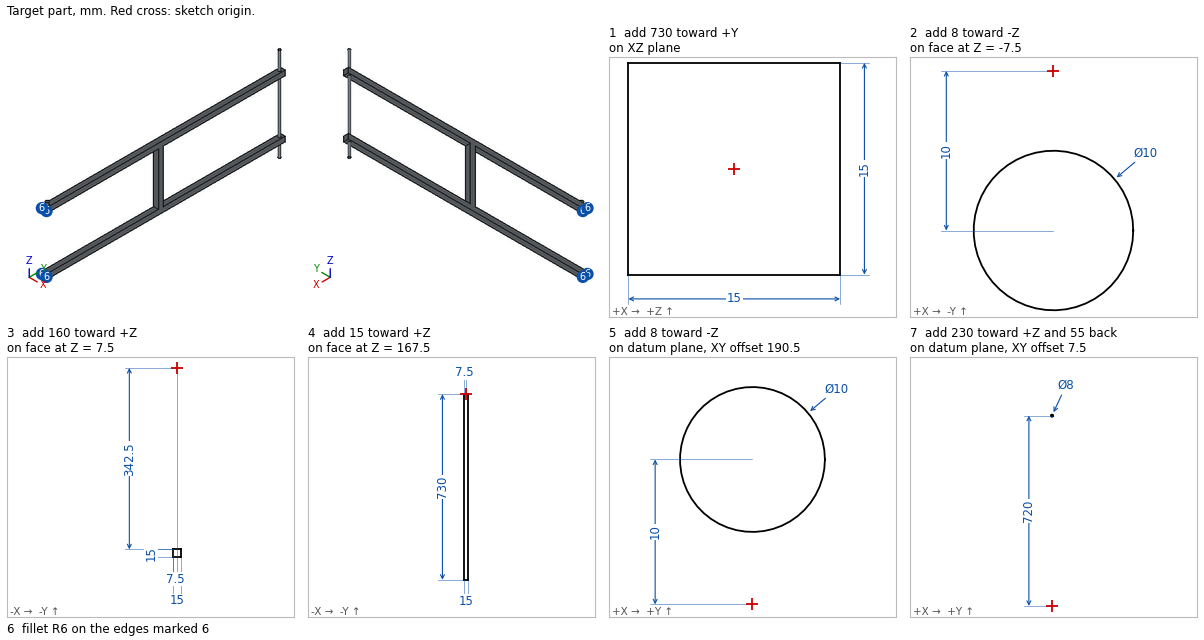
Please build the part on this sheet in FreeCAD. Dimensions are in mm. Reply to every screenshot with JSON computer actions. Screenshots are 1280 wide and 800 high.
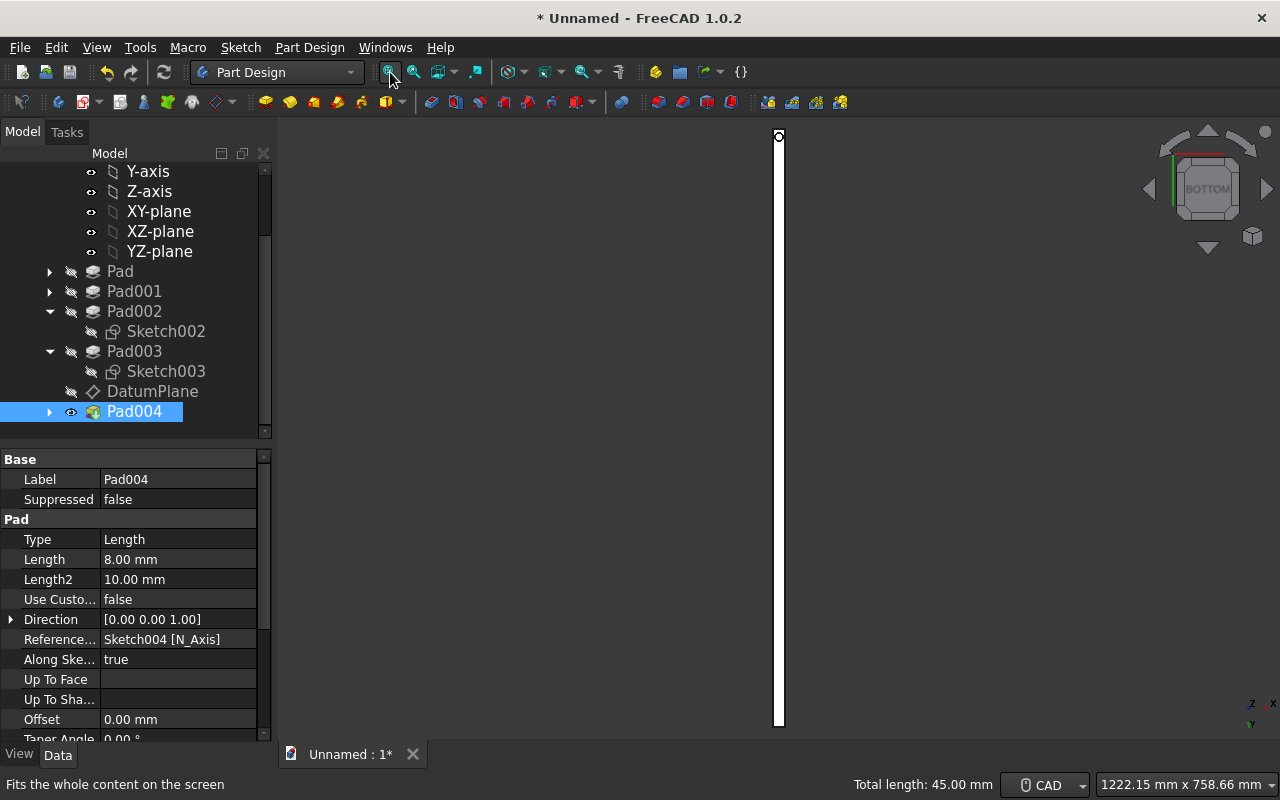
{"action": "key", "text": "4"}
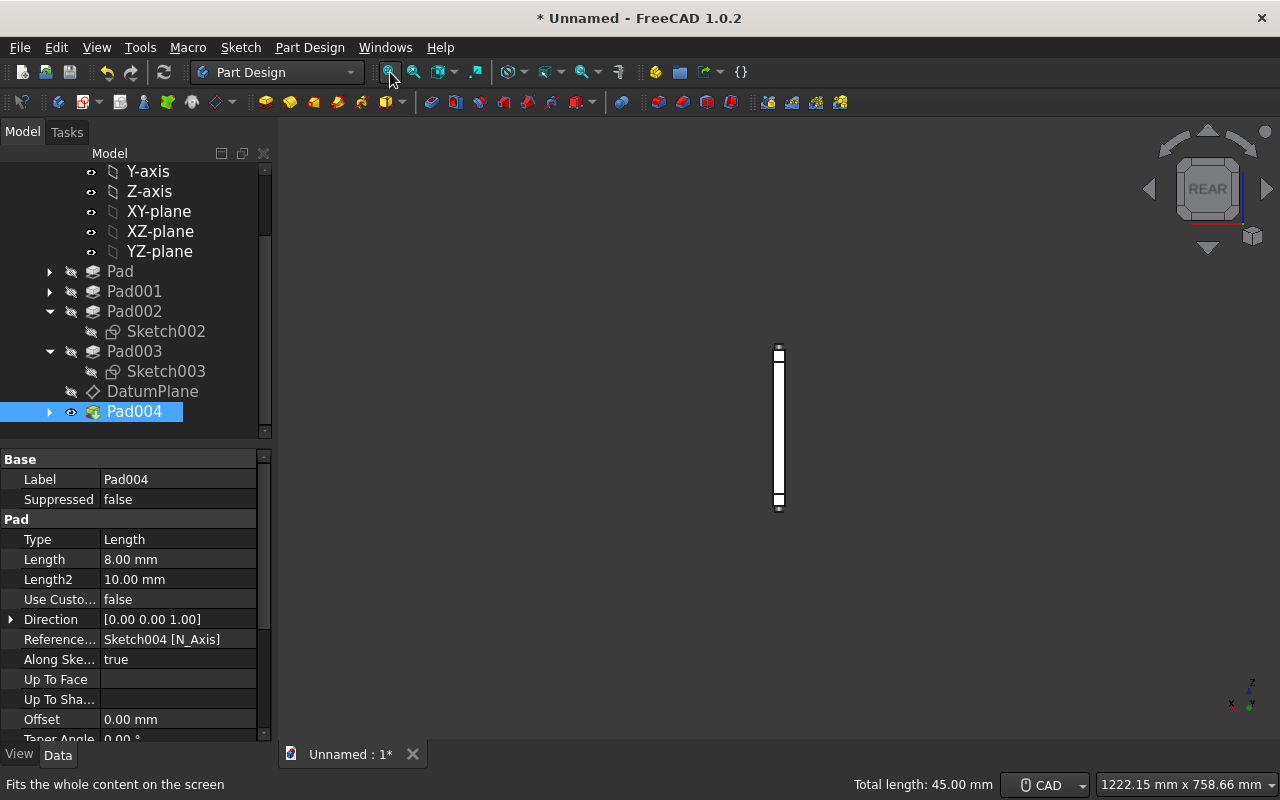
{"action": "left_click", "coordinate": [390, 72]}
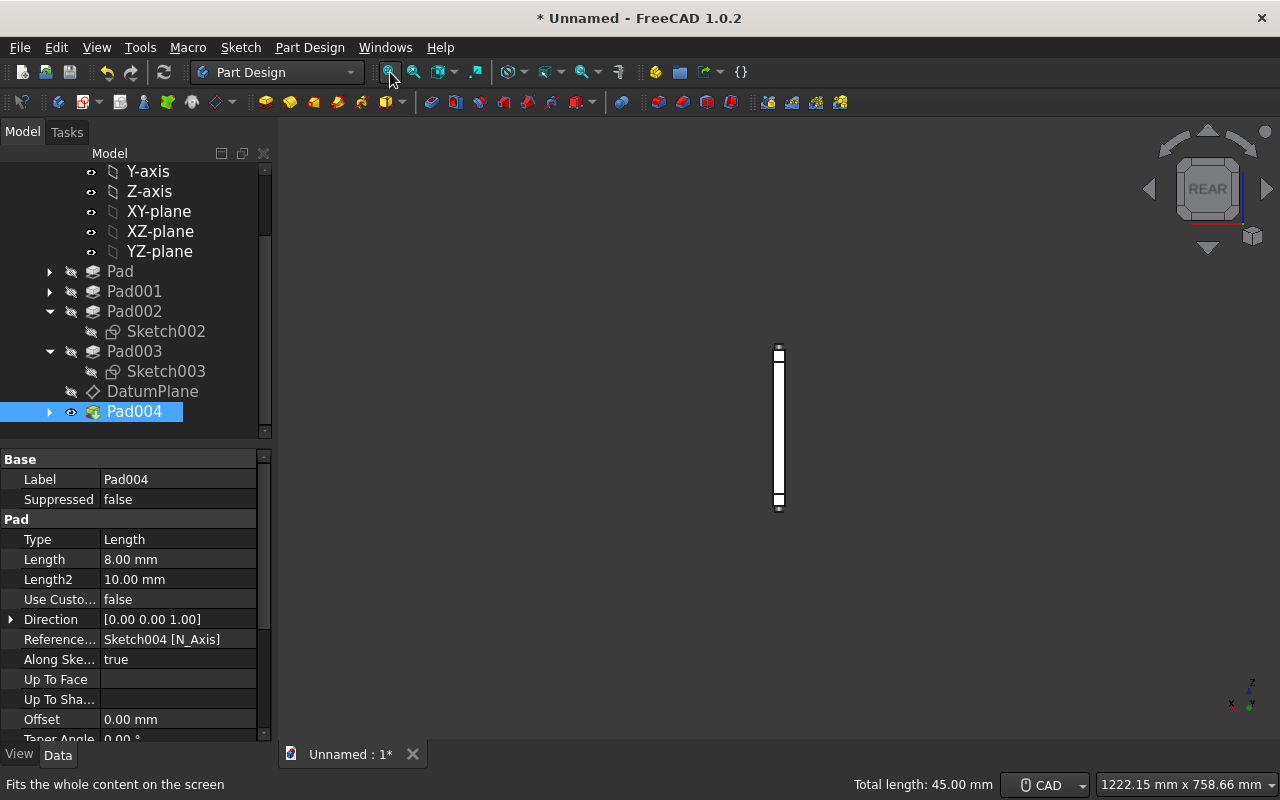
{"action": "scroll", "coordinate": [785, 499], "scroll_direction": "up", "scroll_amount": 6}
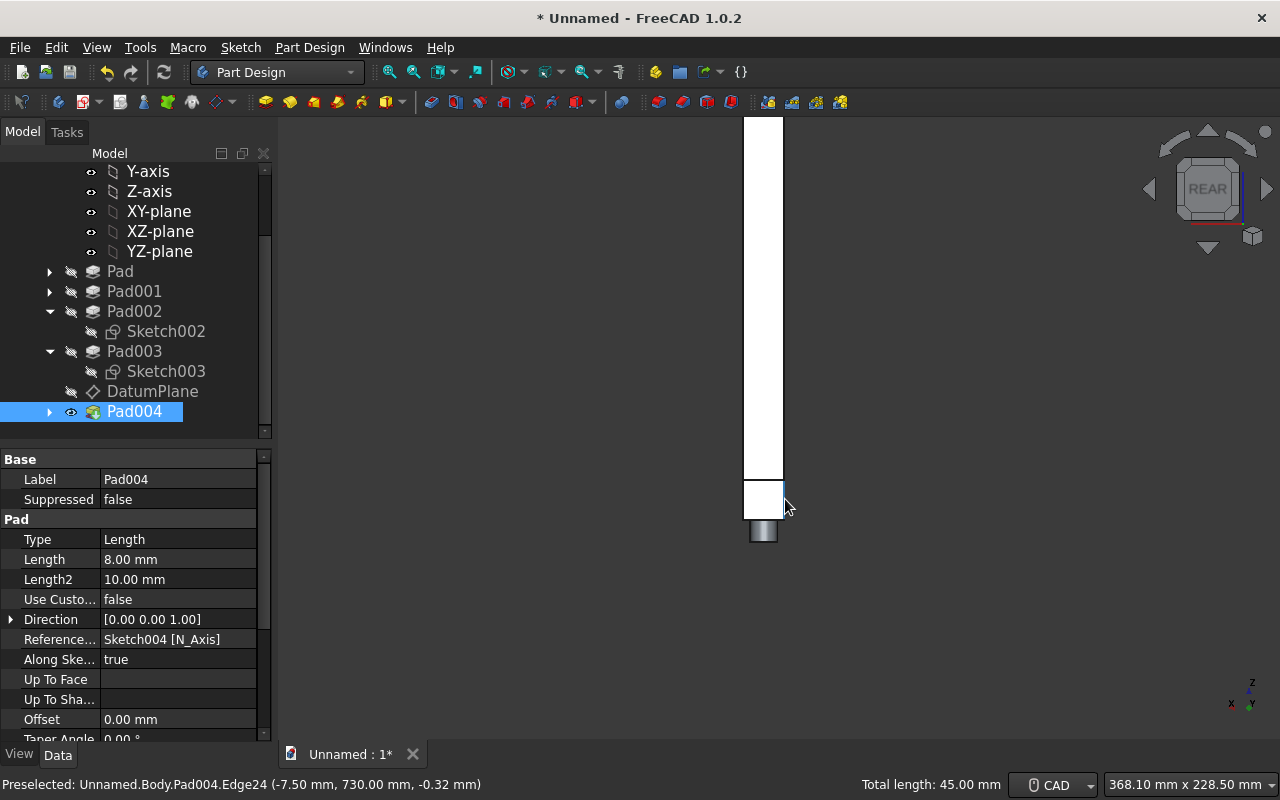
{"action": "left_click", "coordinate": [390, 72]}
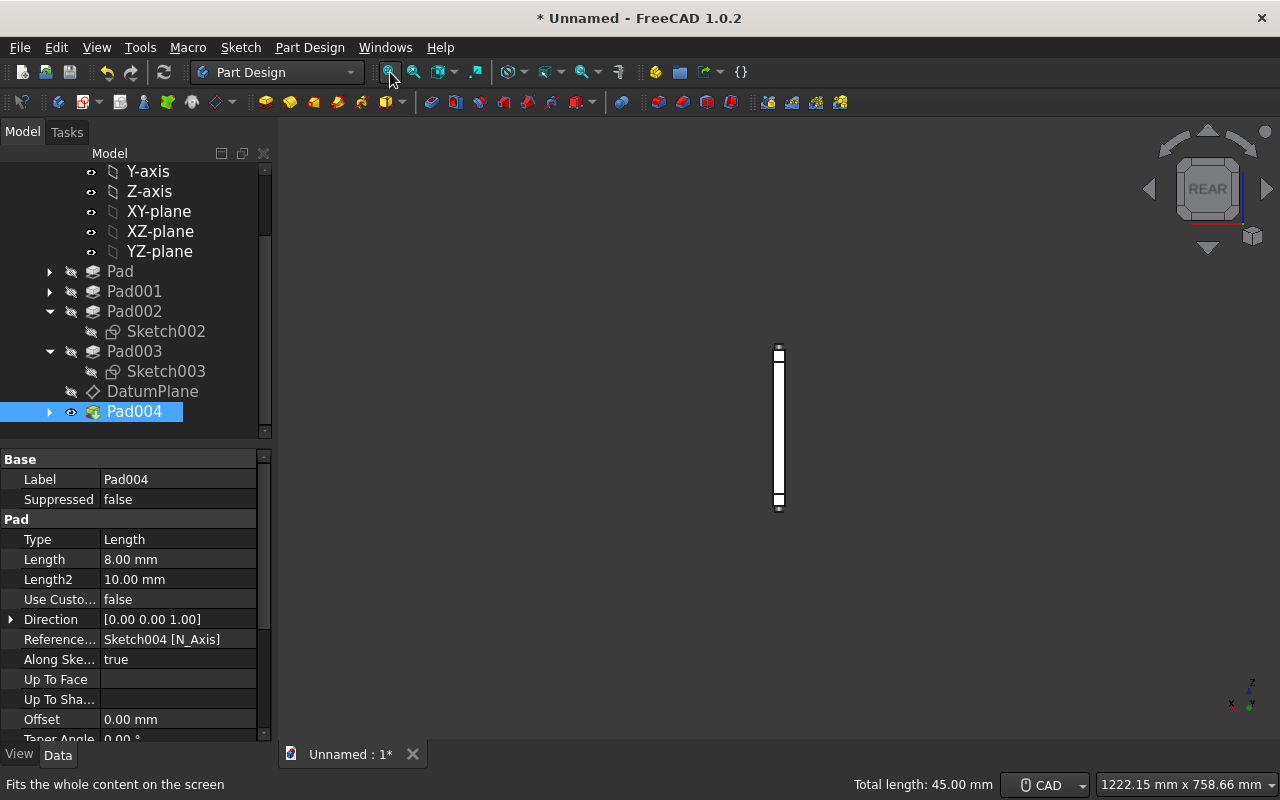
{"action": "key", "text": "6"}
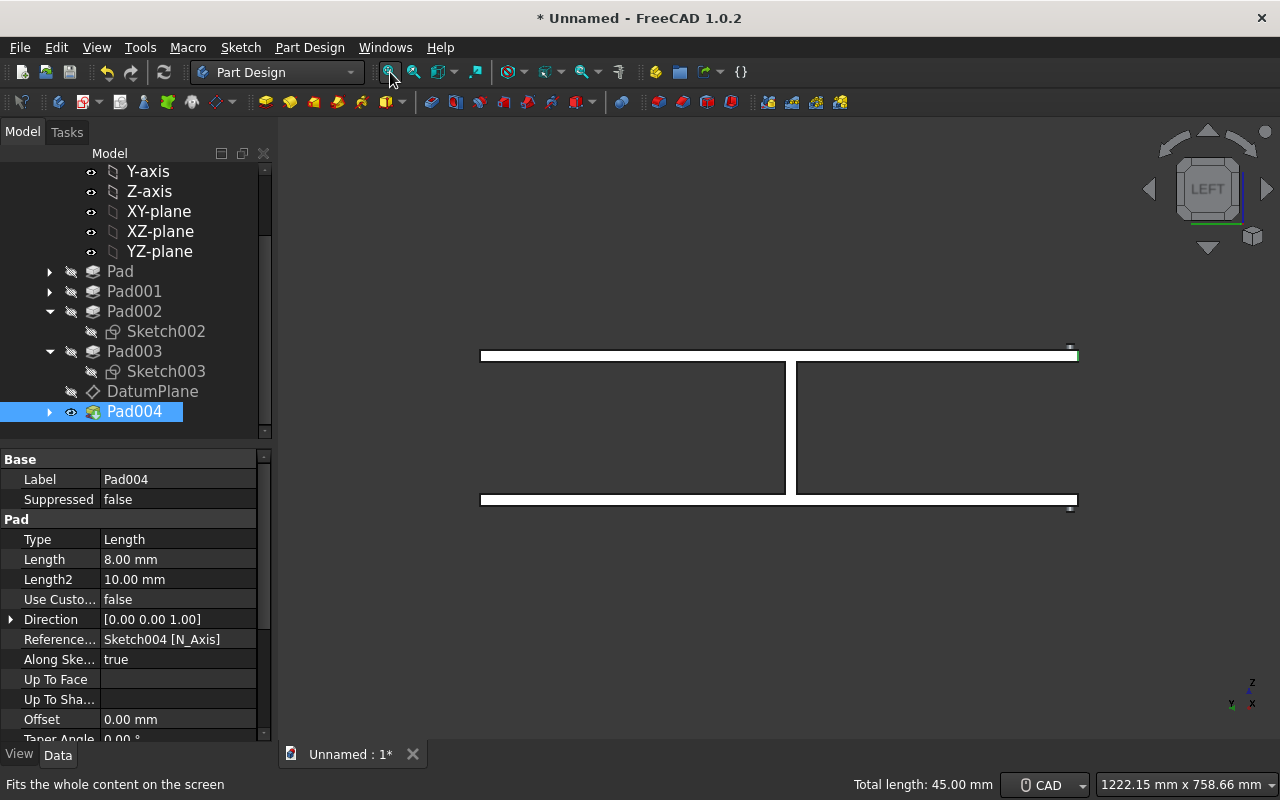
{"action": "scroll", "coordinate": [1078, 499], "scroll_direction": "up", "scroll_amount": 6}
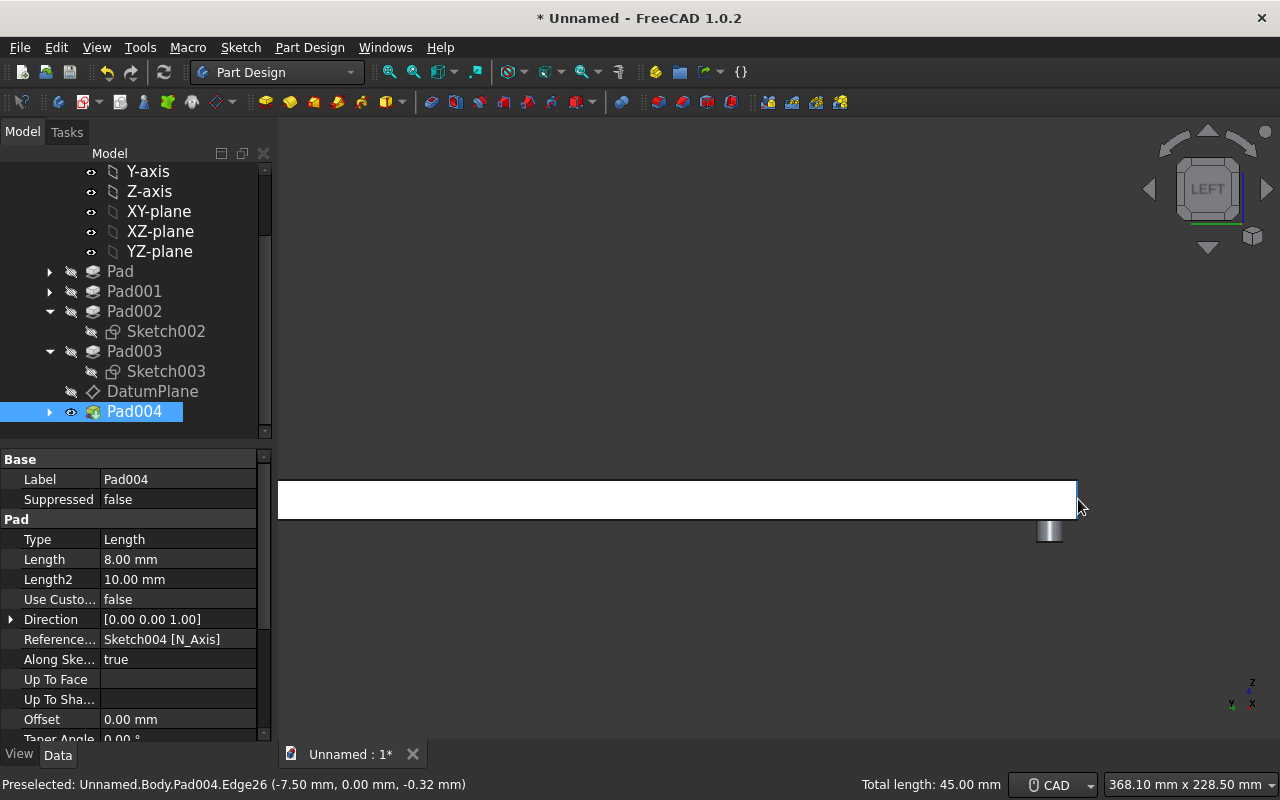
{"action": "left_click", "coordinate": [1077, 499], "text": "ctrl"}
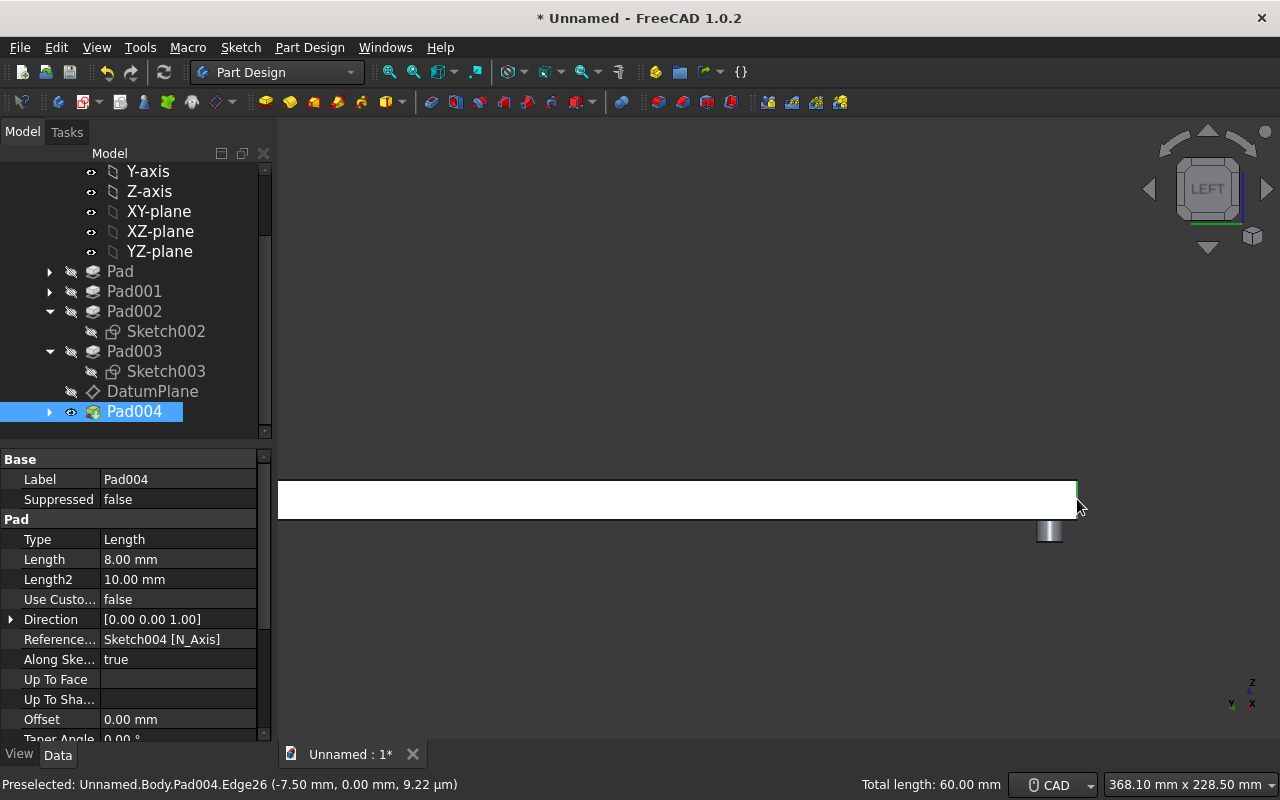
{"action": "left_click", "coordinate": [660, 102]}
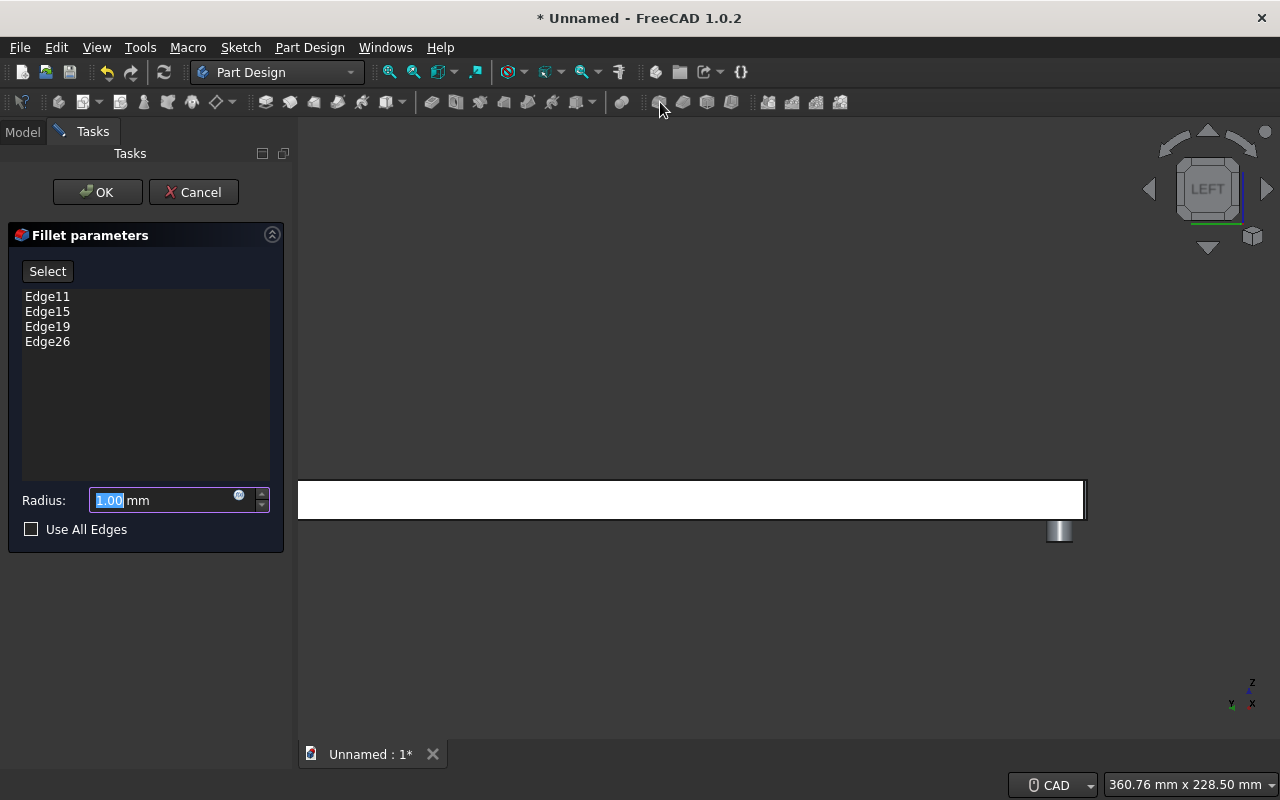
{"action": "type", "text": "6"}
{"action": "key", "text": "Tab"}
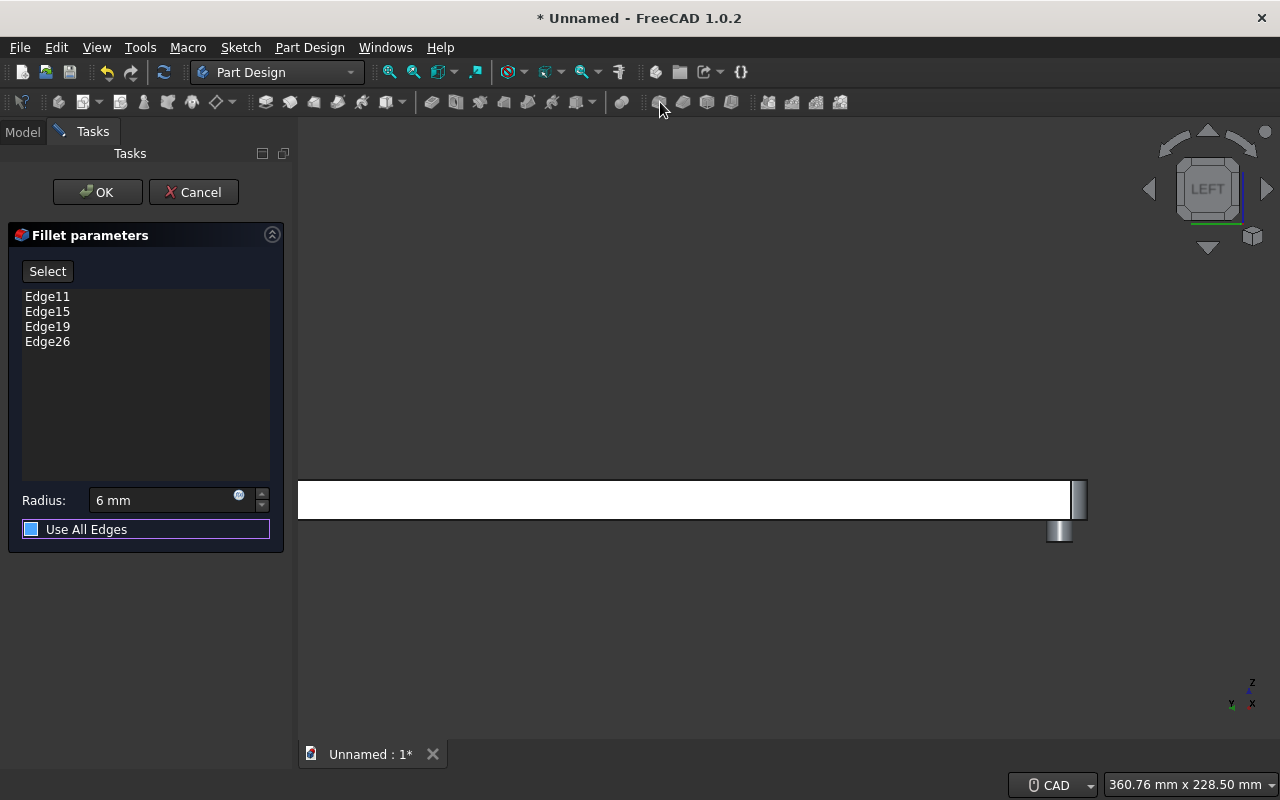
{"action": "left_click", "coordinate": [98, 192]}